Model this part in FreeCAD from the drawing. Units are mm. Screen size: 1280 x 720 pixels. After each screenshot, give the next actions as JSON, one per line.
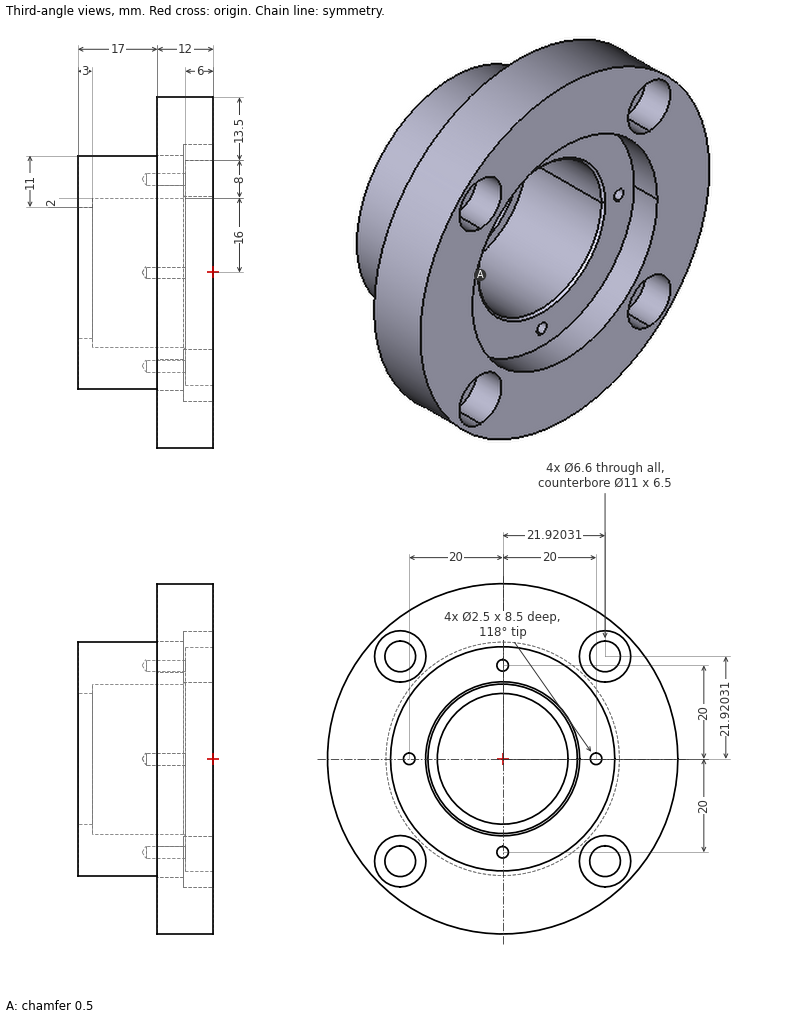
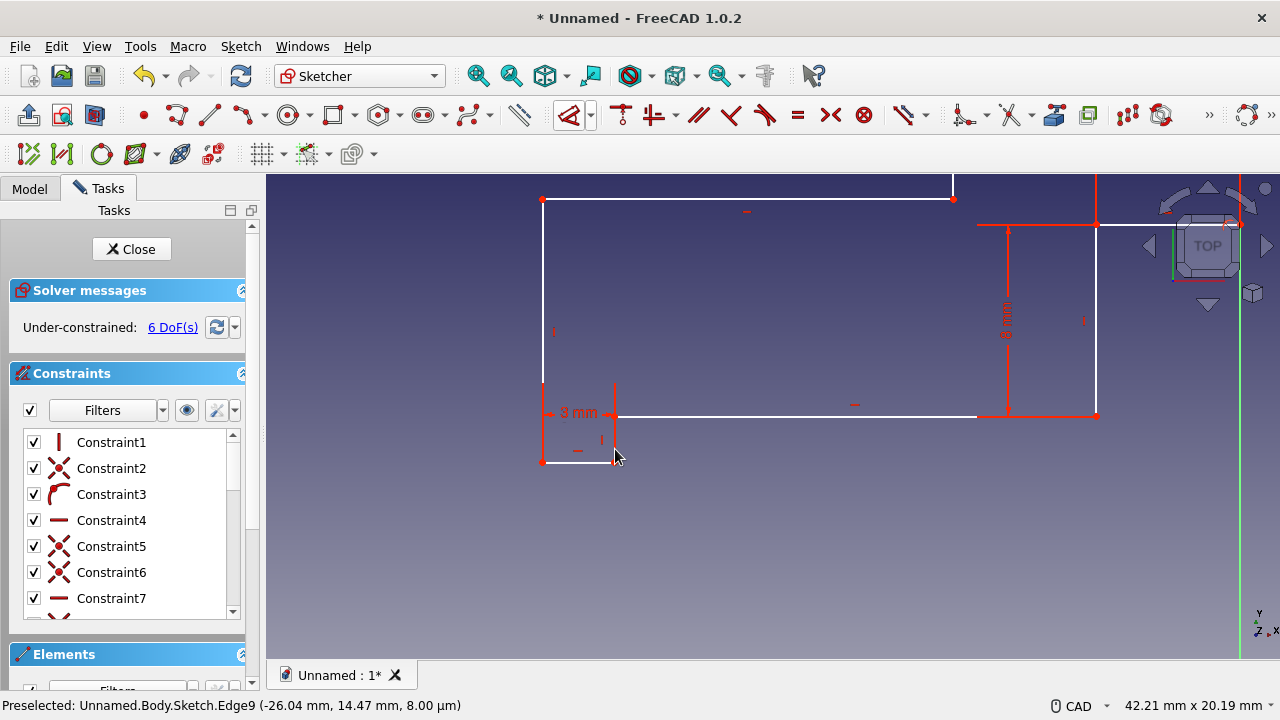
{"action": "key", "text": "i"}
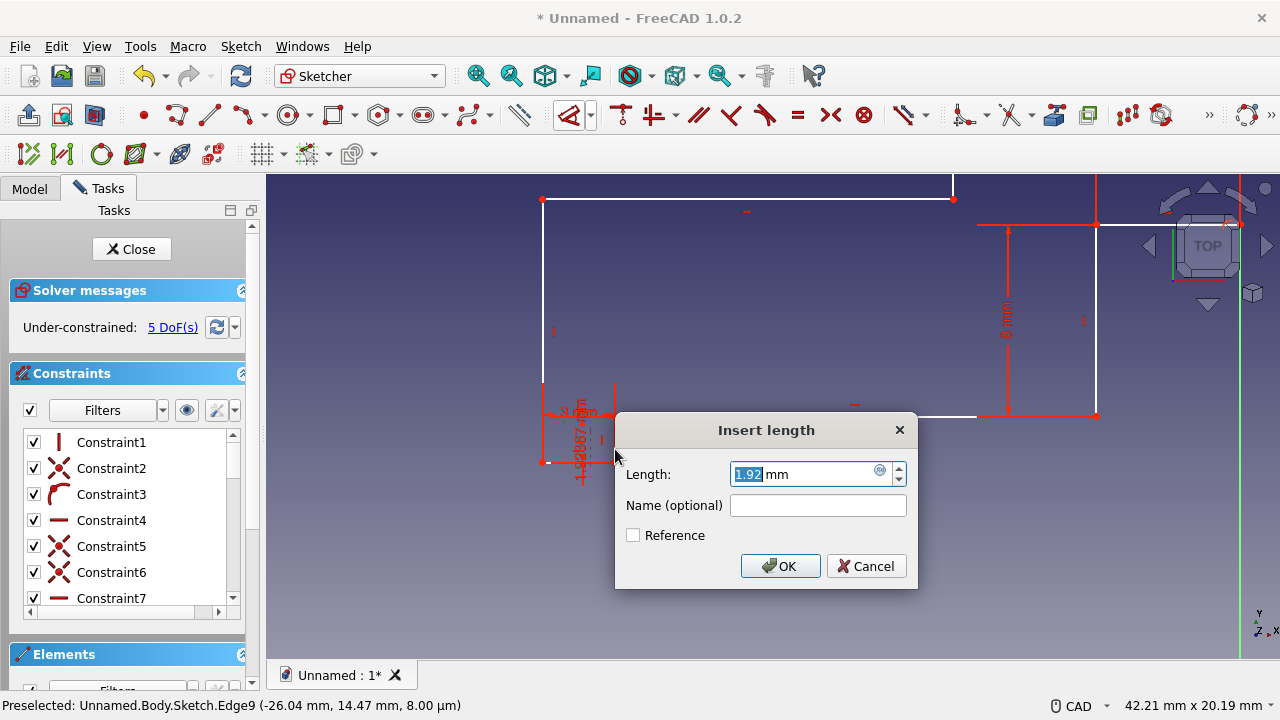
{"action": "type", "text": "2"}
{"action": "key", "text": "Return"}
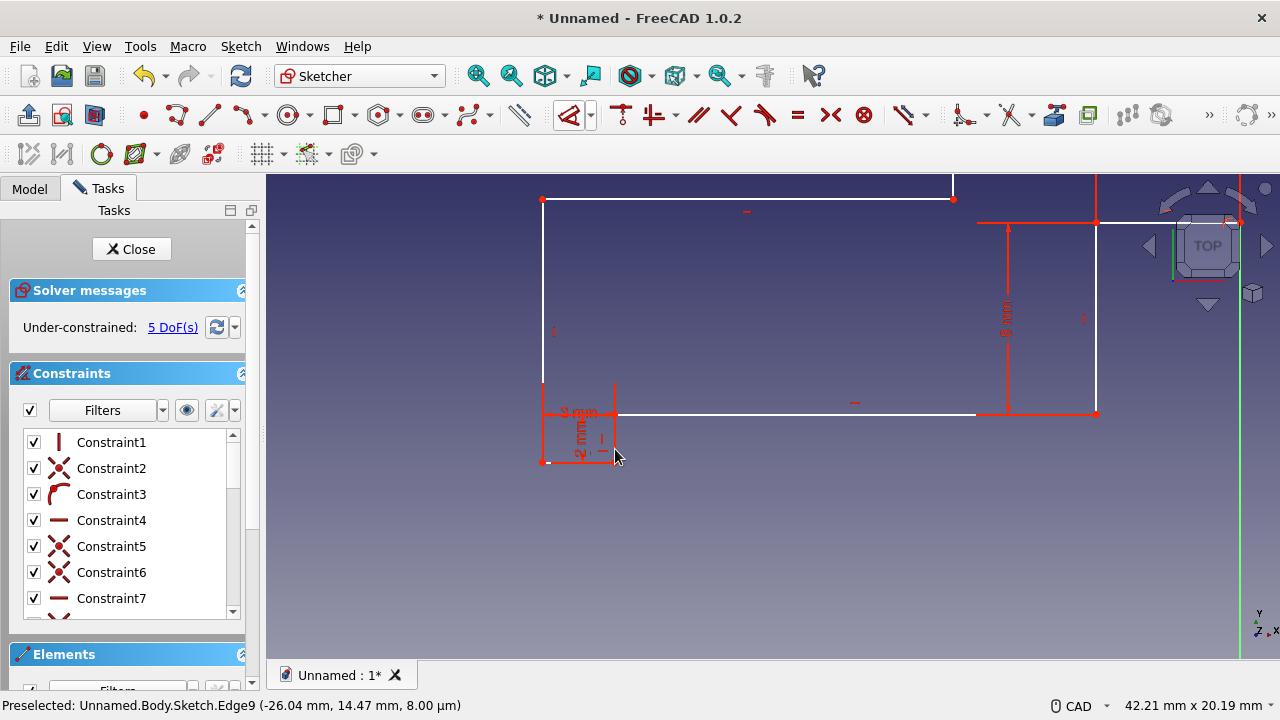
{"action": "scroll", "coordinate": [595, 457], "scroll_direction": "down", "scroll_amount": 5}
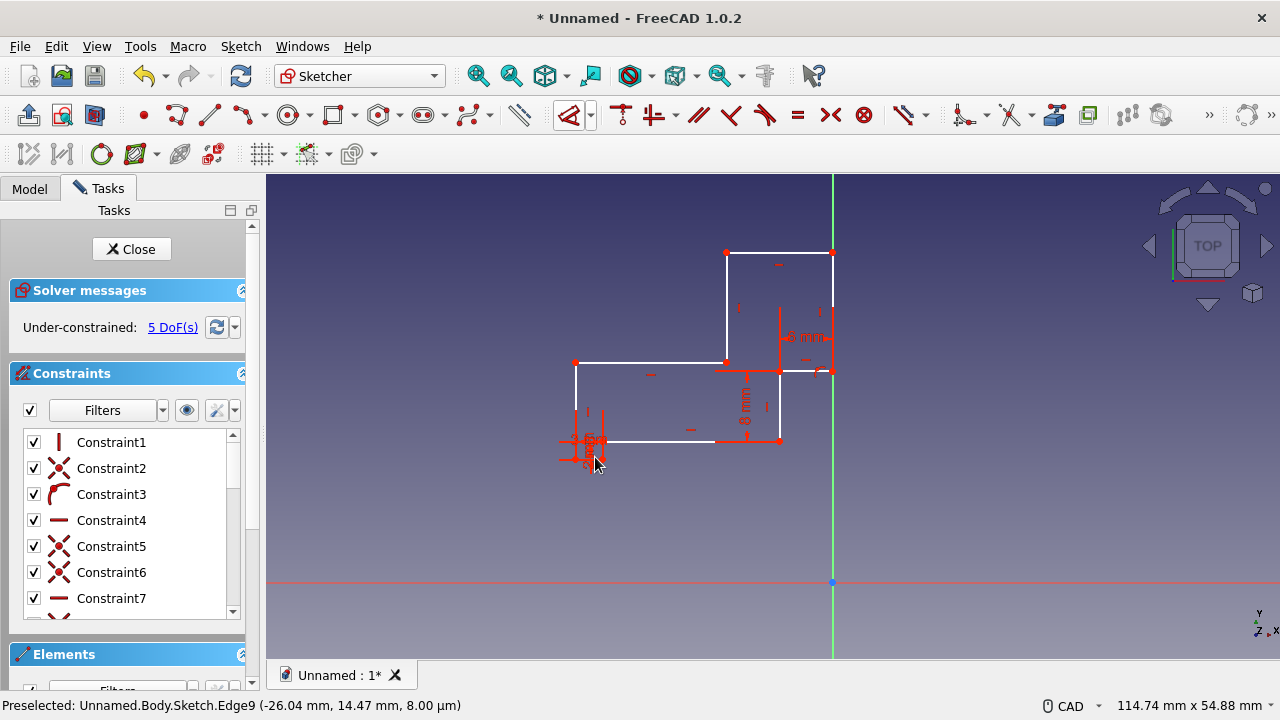
{"action": "left_click", "coordinate": [801, 253]}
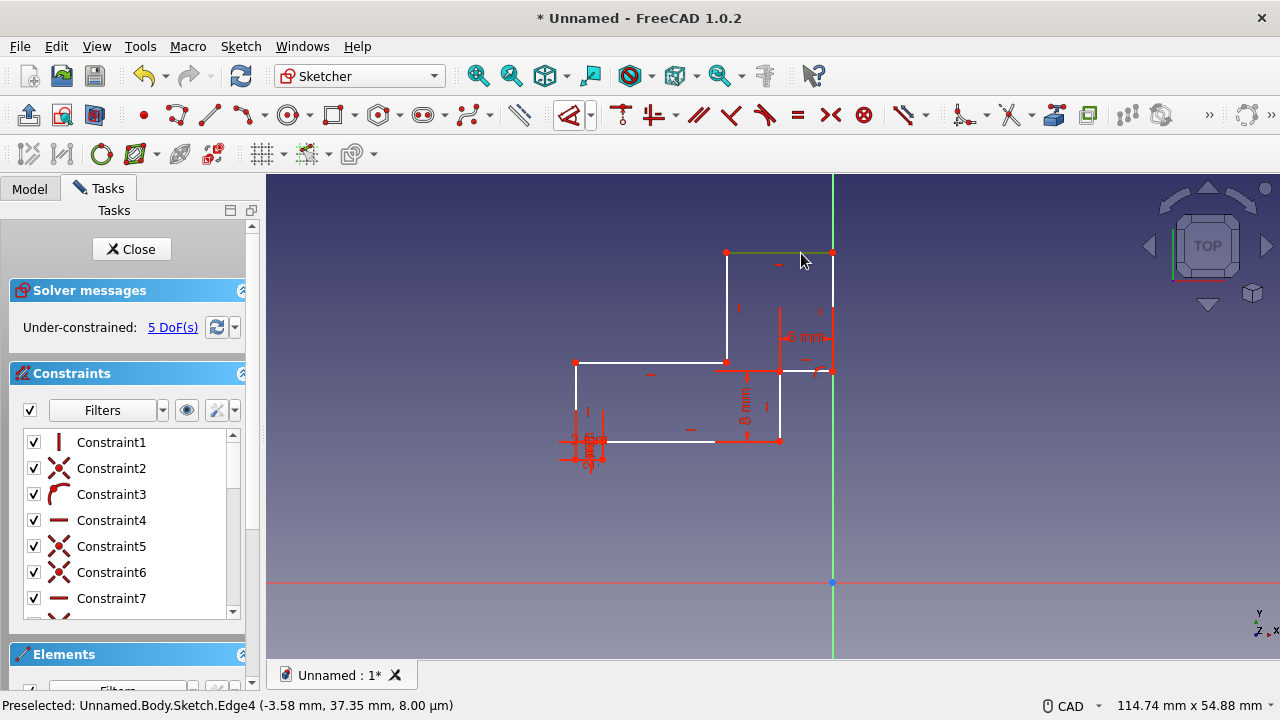
{"action": "key", "text": "l"}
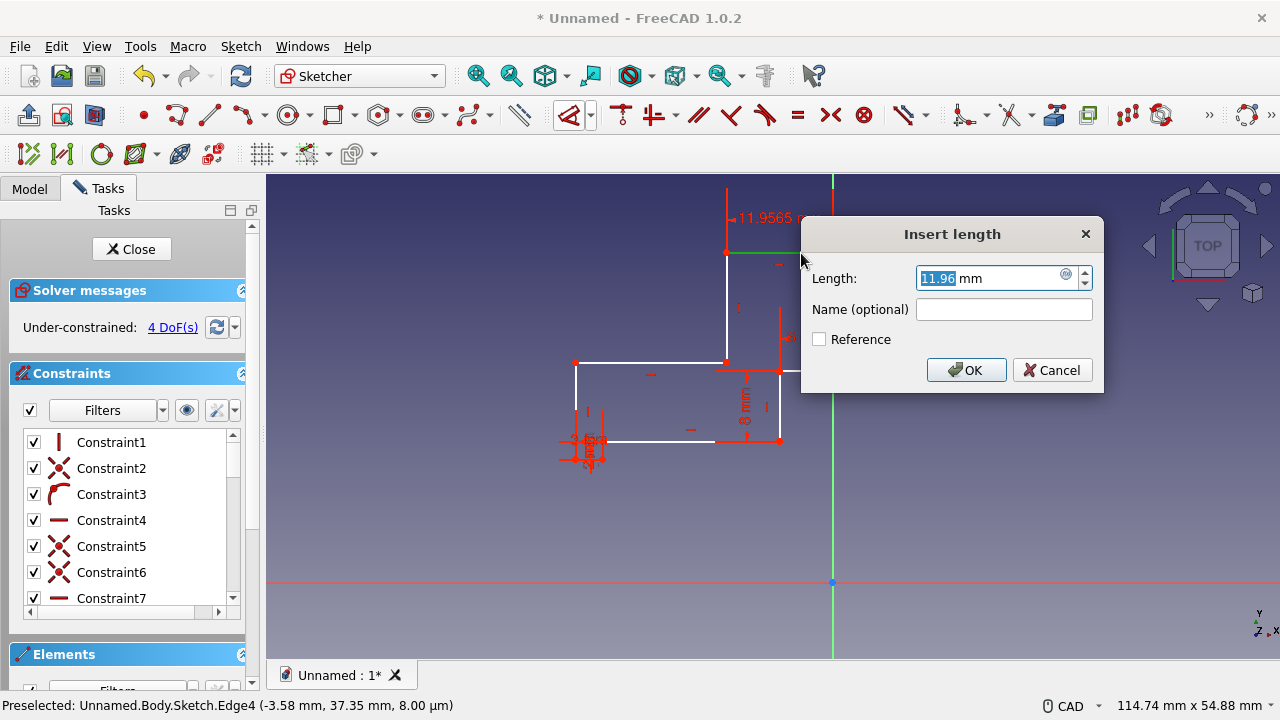
{"action": "type", "text": "12"}
{"action": "key", "text": "Return"}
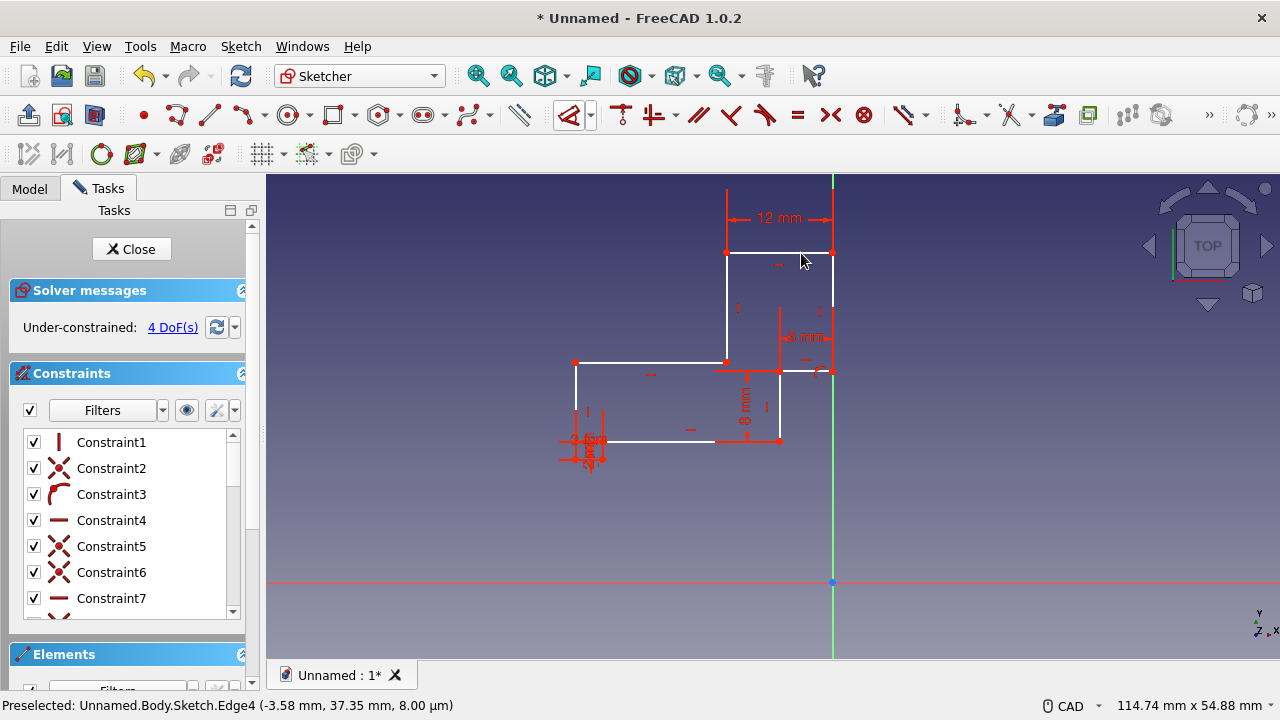
{"action": "left_click", "coordinate": [681, 363]}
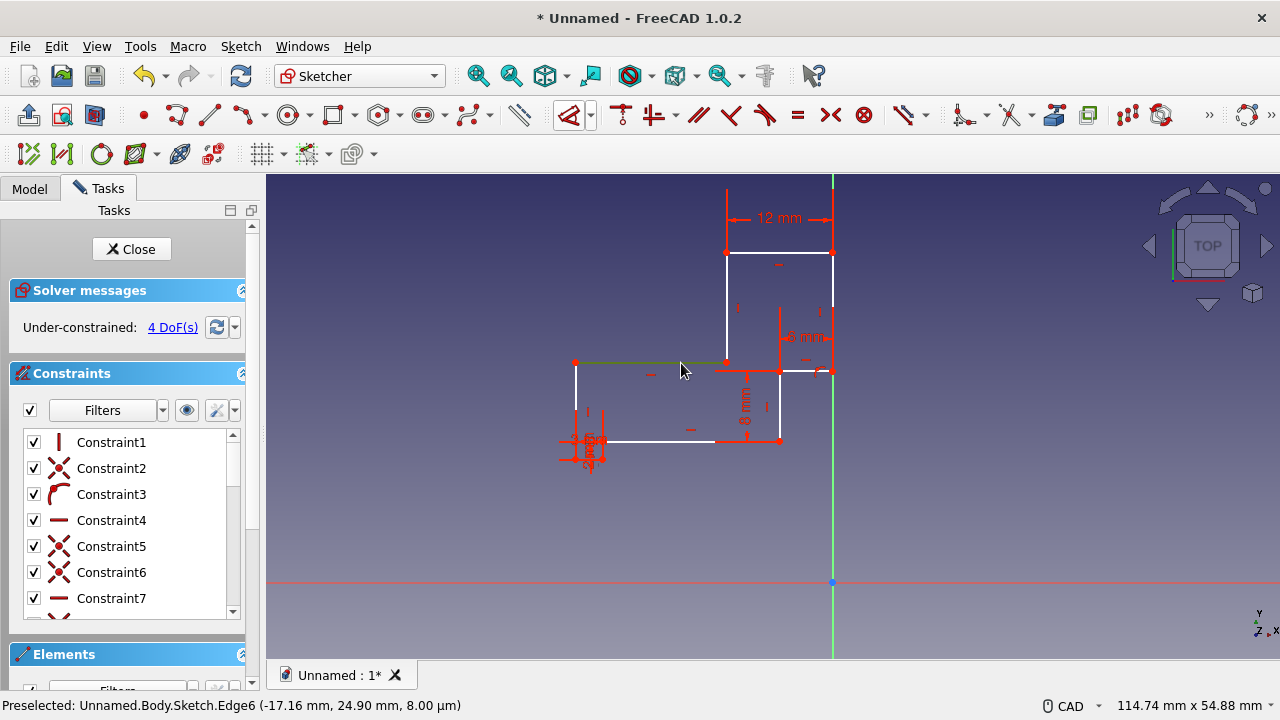
{"action": "key", "text": "l"}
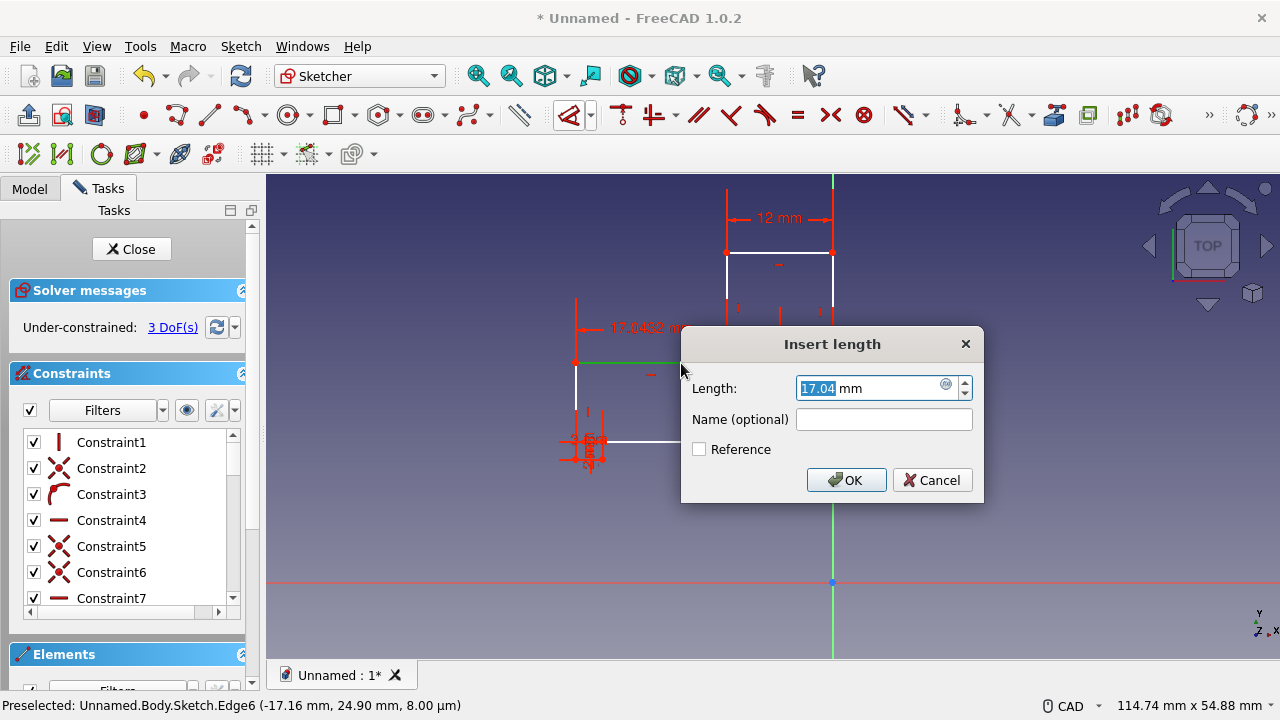
{"action": "type", "text": "17"}
{"action": "key", "text": "Return"}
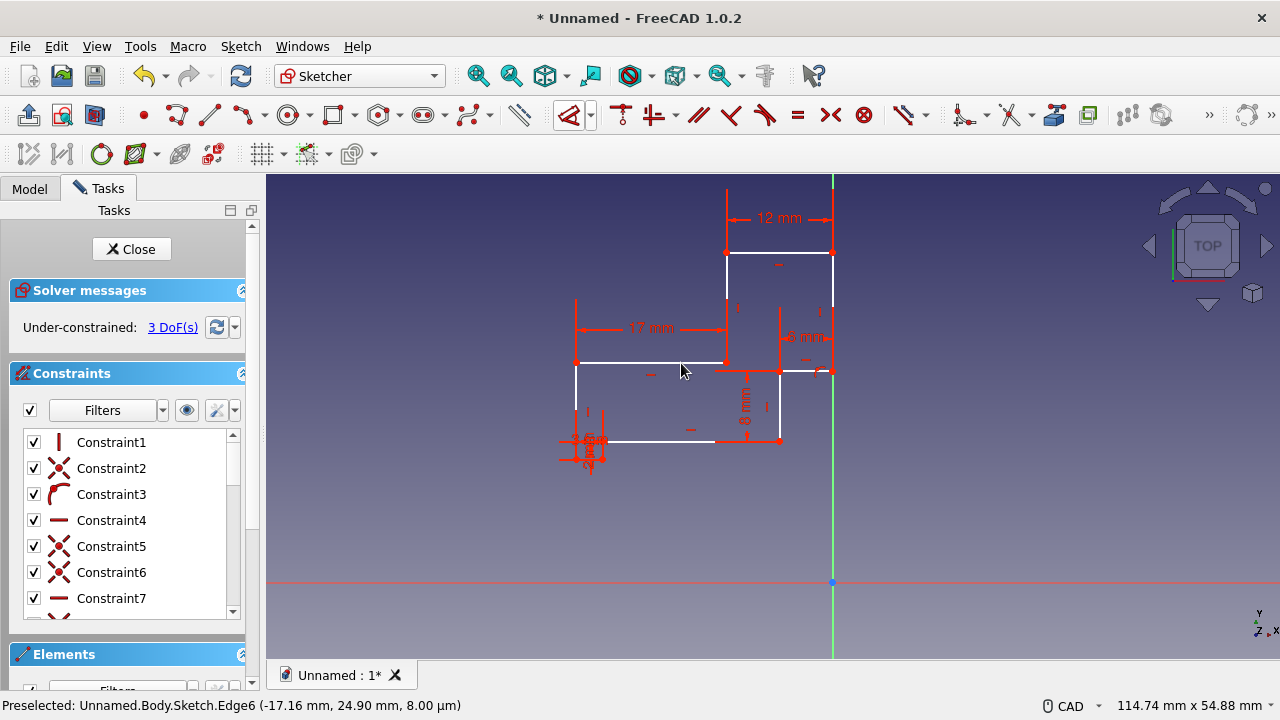
{"action": "left_click", "coordinate": [576, 392]}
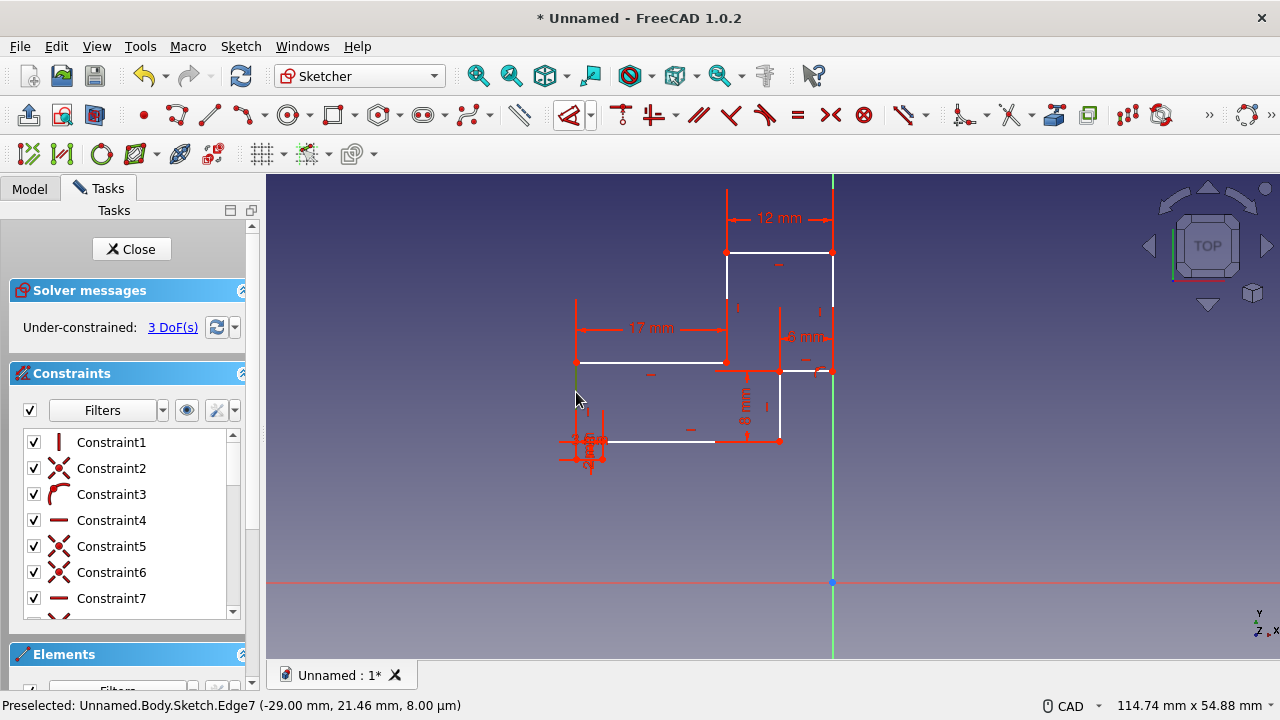
{"action": "left_click", "coordinate": [590, 116]}